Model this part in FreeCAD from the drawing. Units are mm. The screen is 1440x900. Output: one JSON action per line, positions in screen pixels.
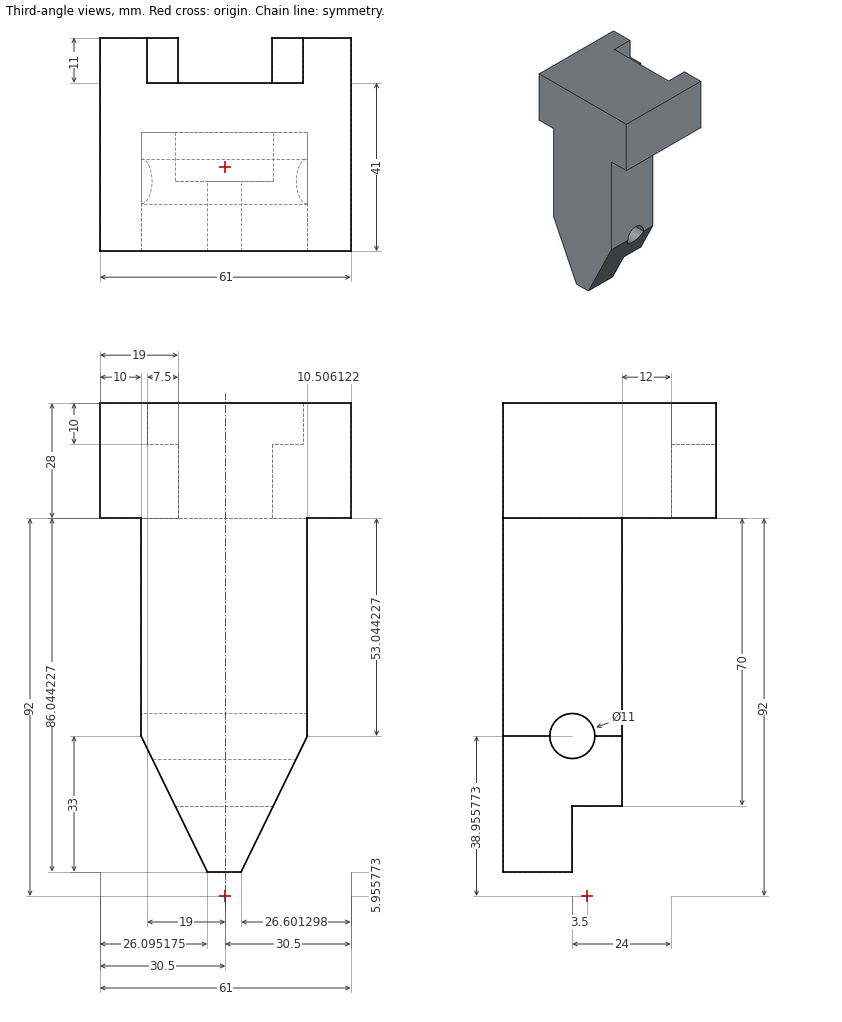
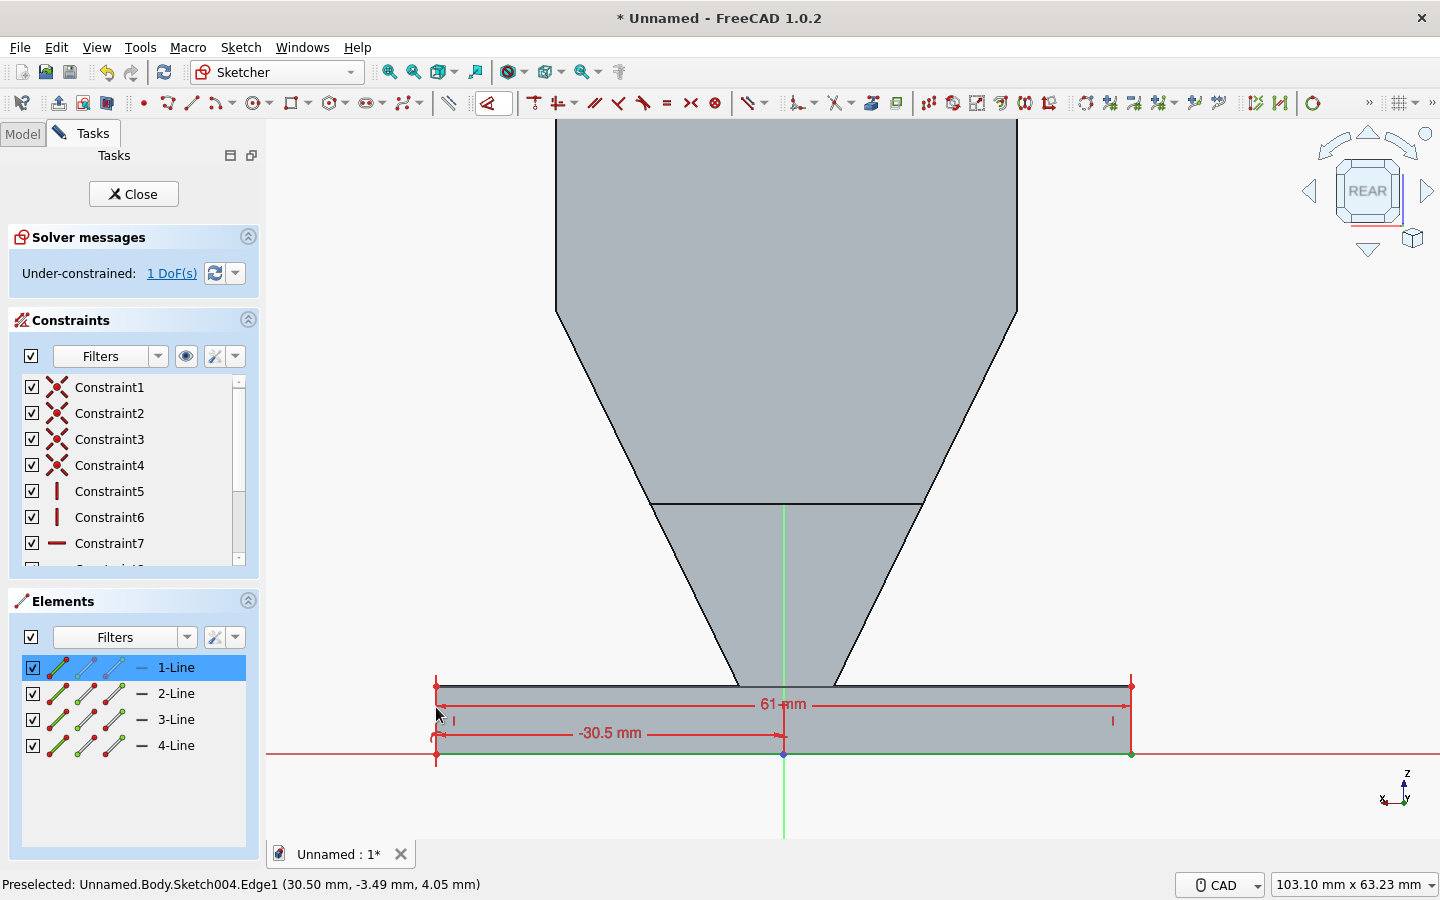
{"action": "key", "text": "i"}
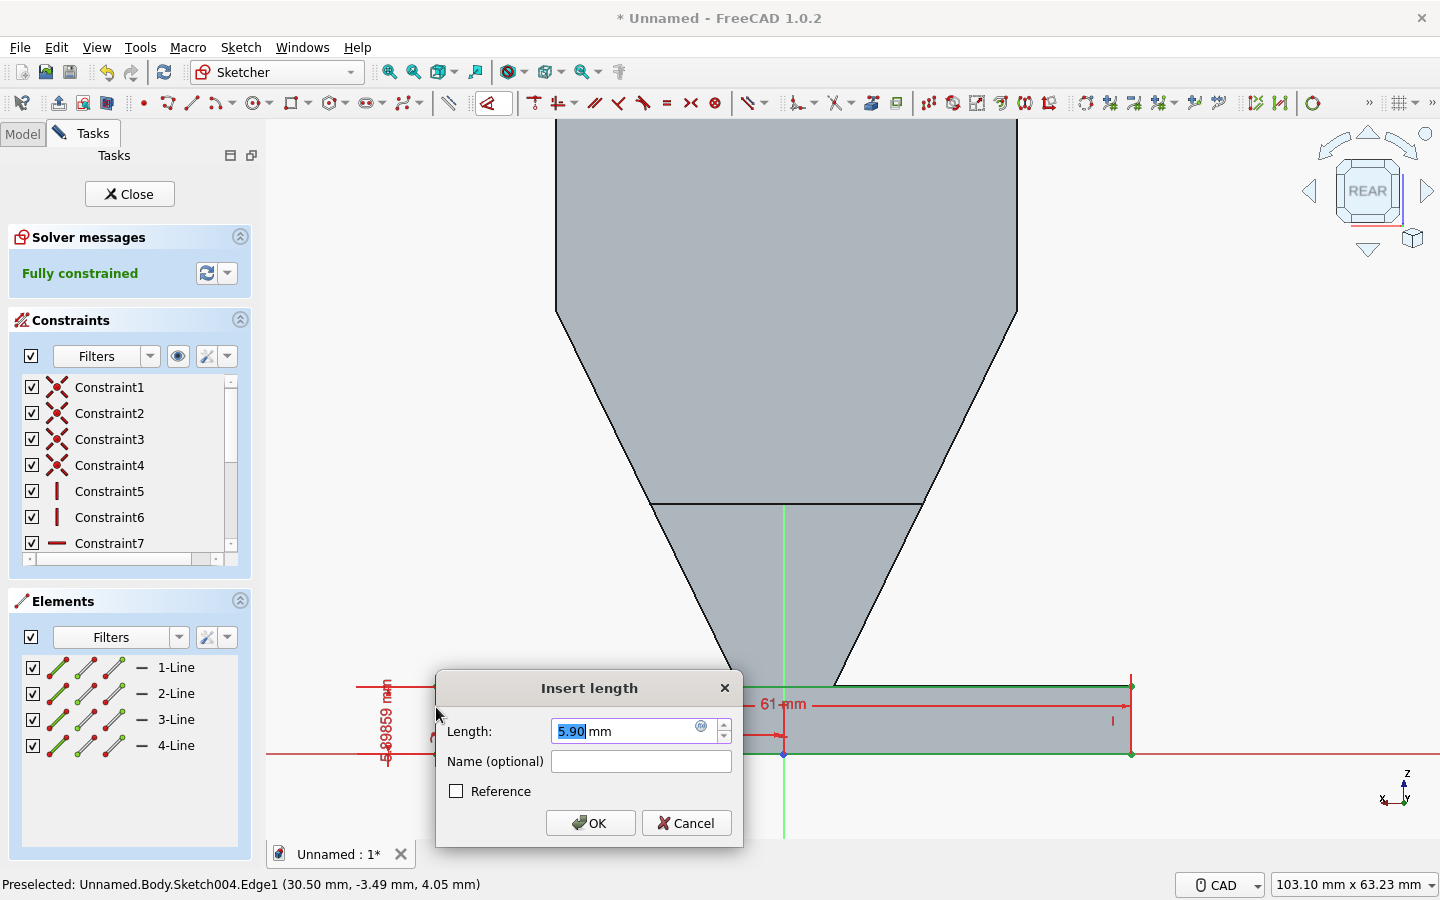
{"action": "type", "text": "5.955773"}
{"action": "key", "text": "Return"}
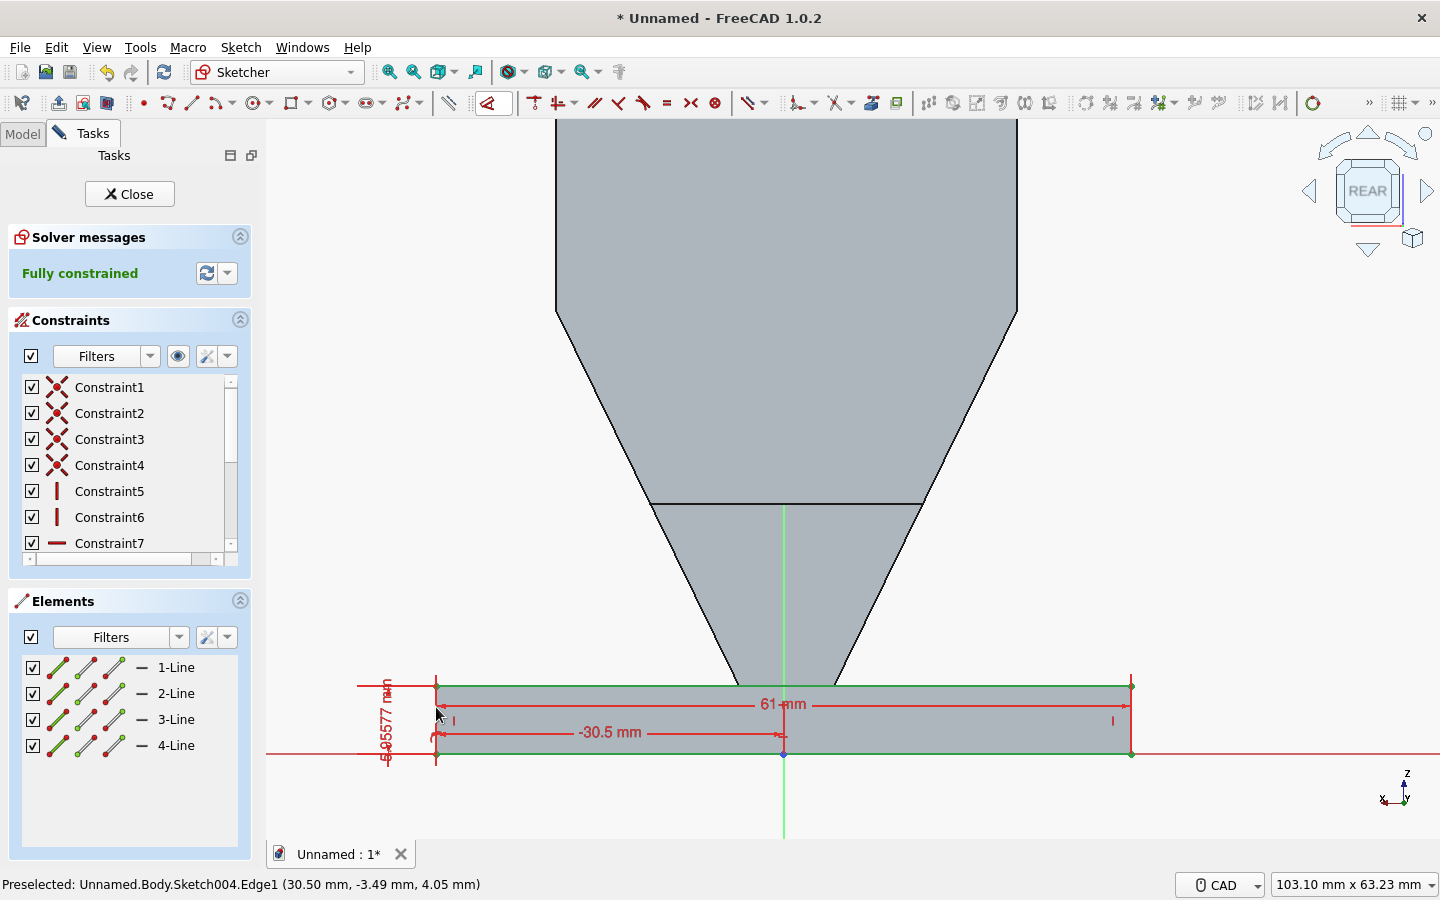
{"action": "left_click", "coordinate": [130, 194]}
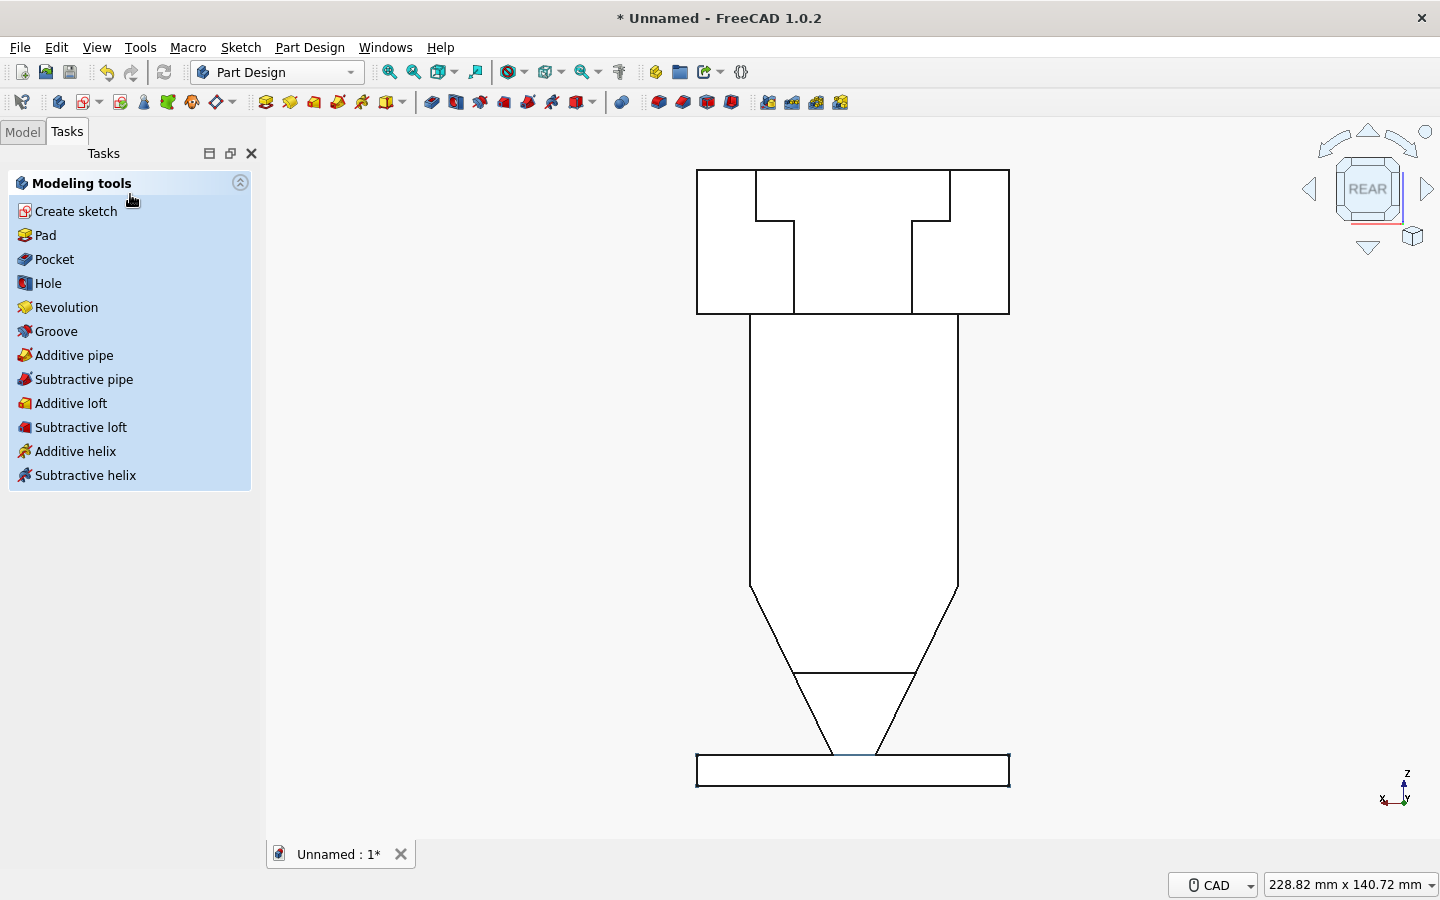
{"action": "left_click", "coordinate": [432, 102]}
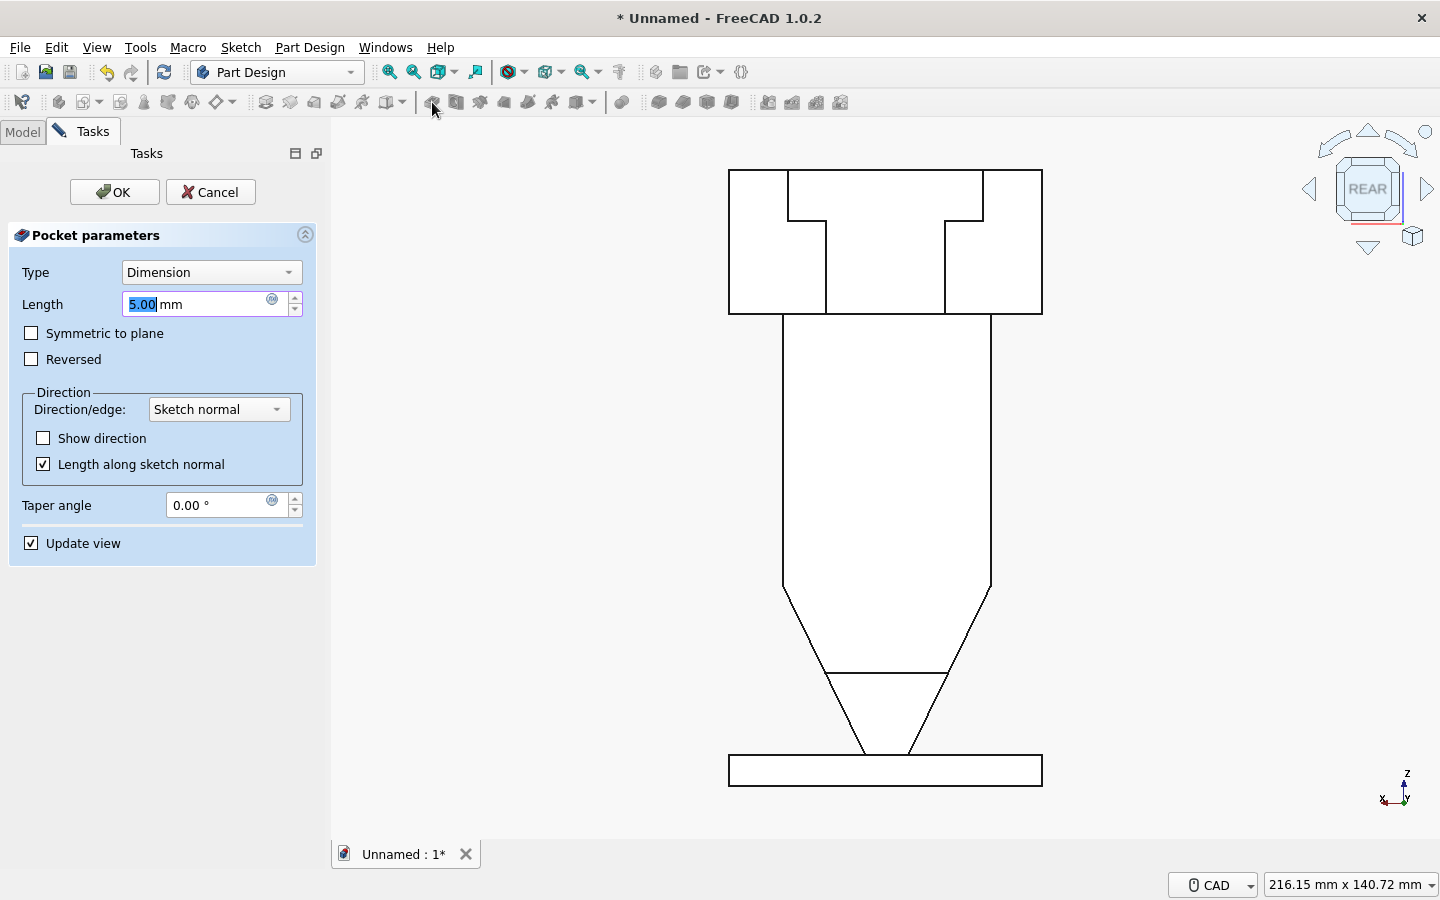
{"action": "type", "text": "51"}
{"action": "key", "text": "Tab"}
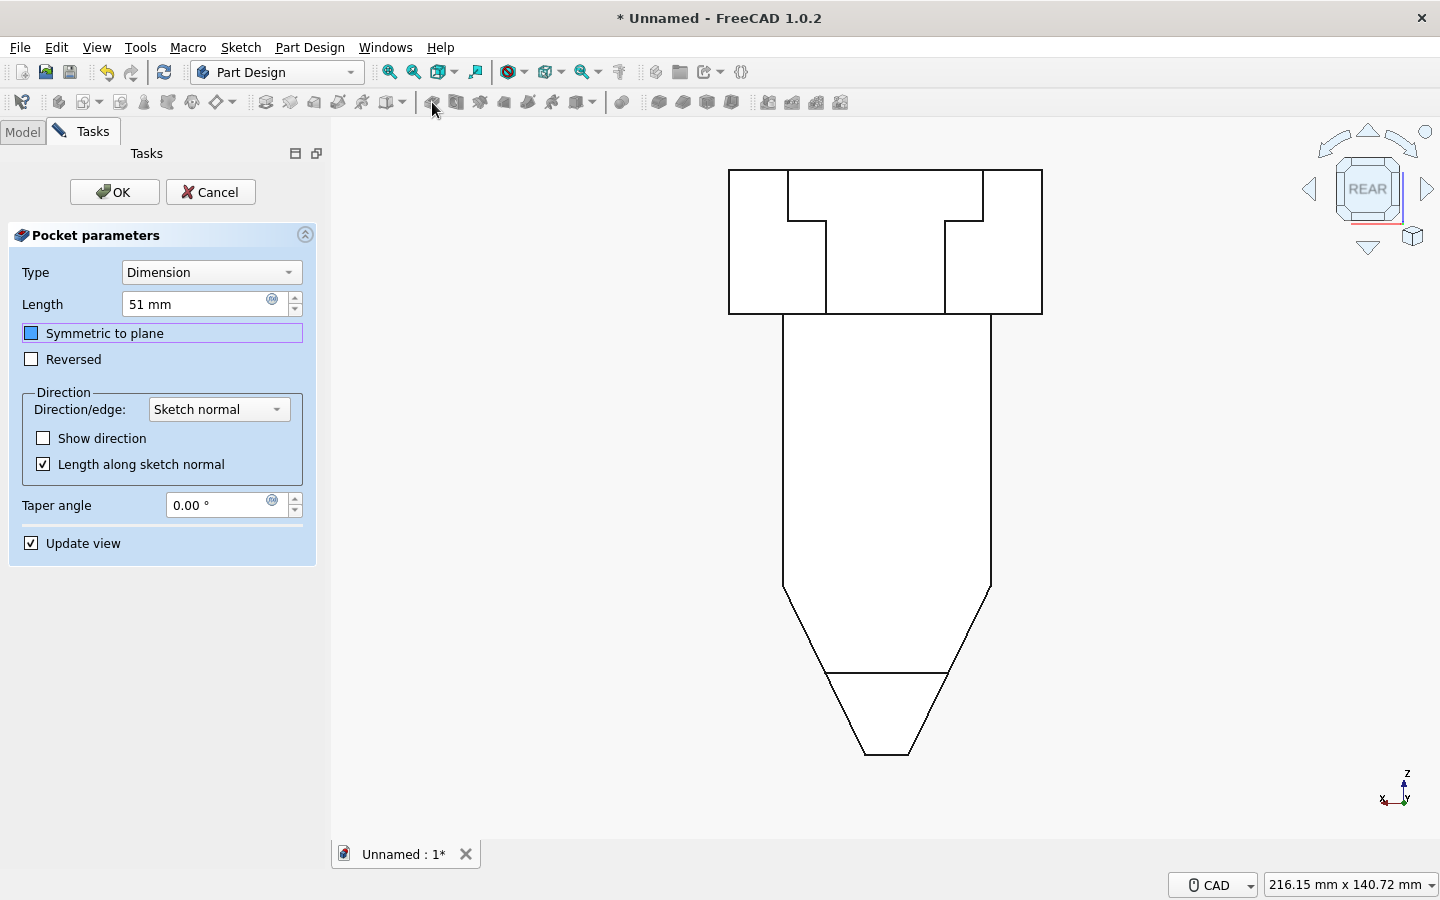
{"action": "left_click", "coordinate": [115, 192]}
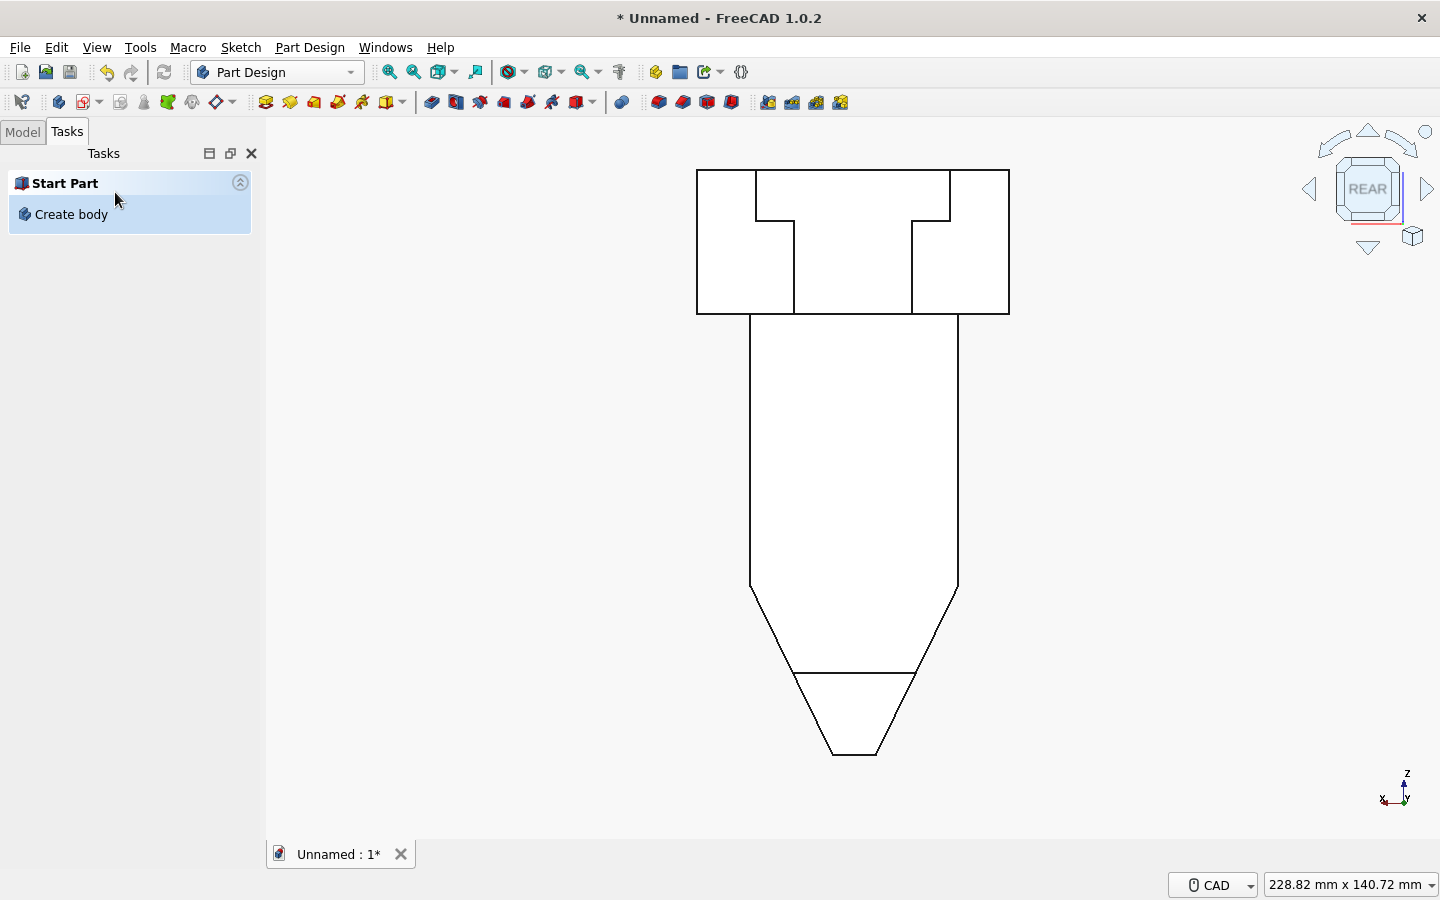
{"action": "left_click", "coordinate": [84, 102]}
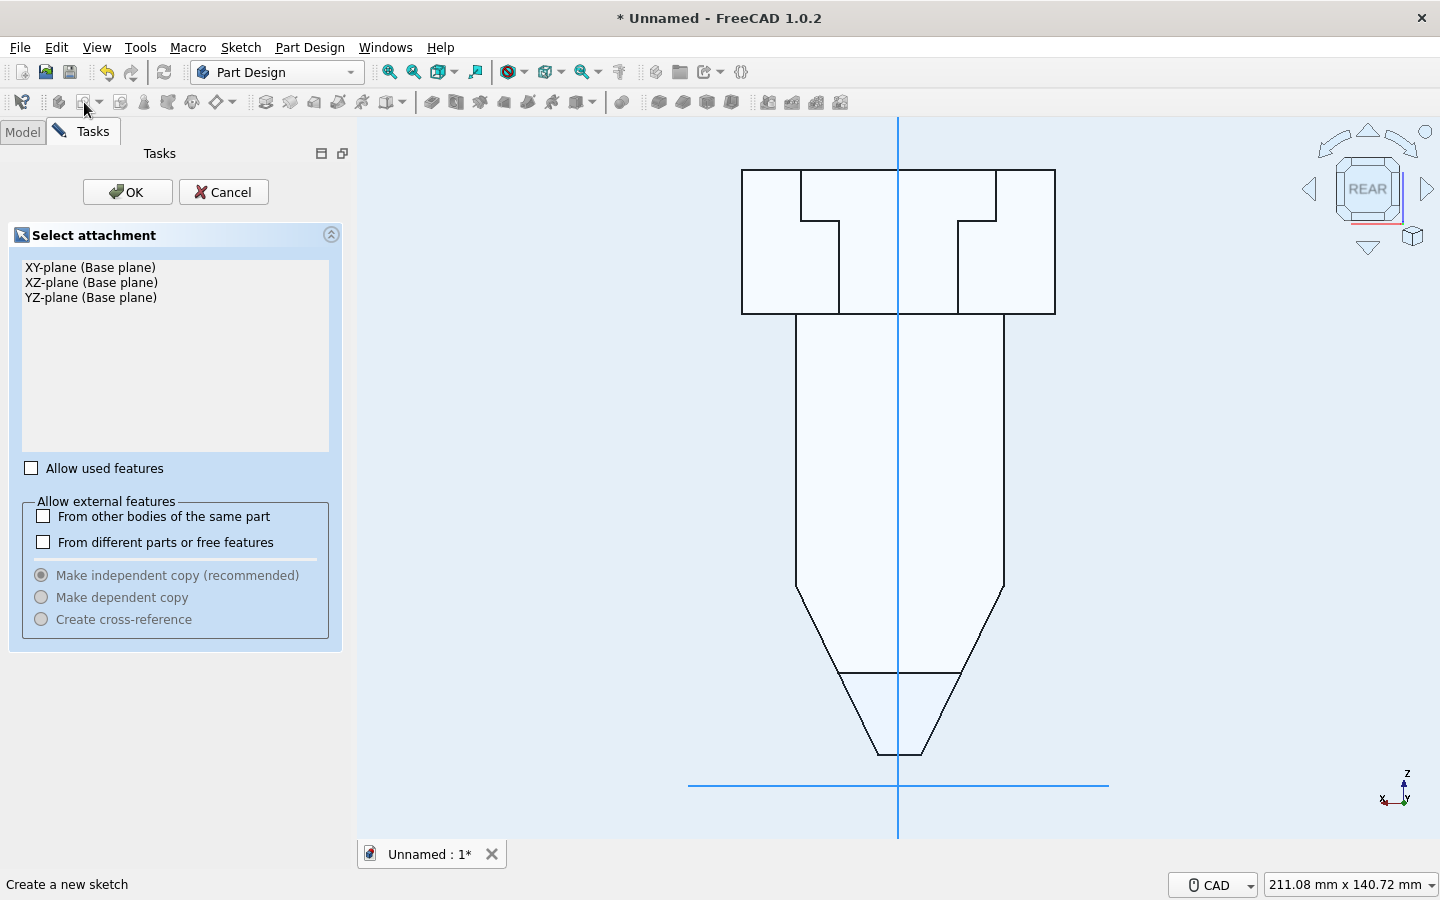
{"action": "left_click", "coordinate": [82, 298]}